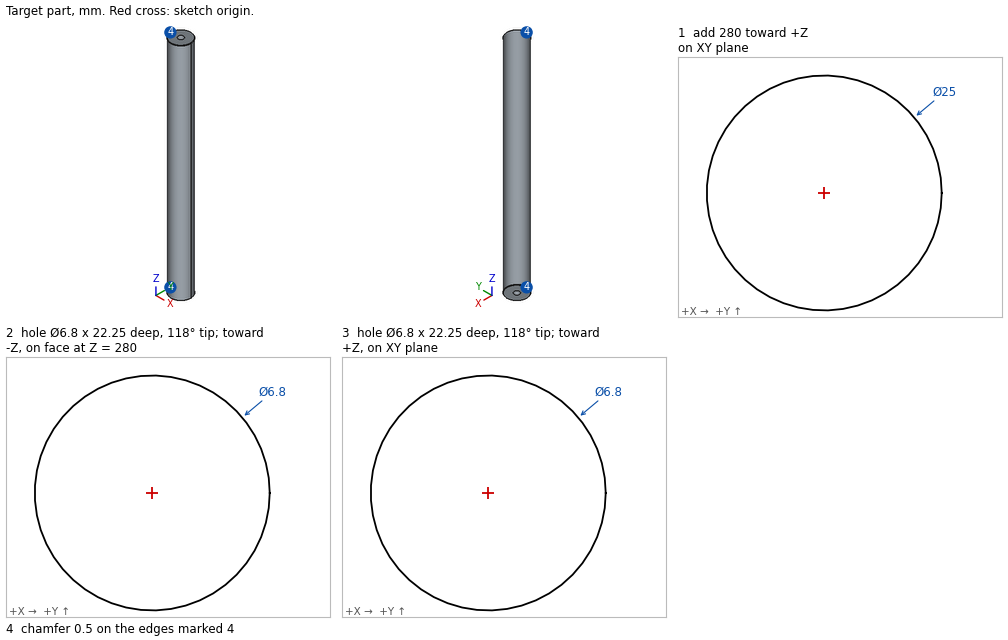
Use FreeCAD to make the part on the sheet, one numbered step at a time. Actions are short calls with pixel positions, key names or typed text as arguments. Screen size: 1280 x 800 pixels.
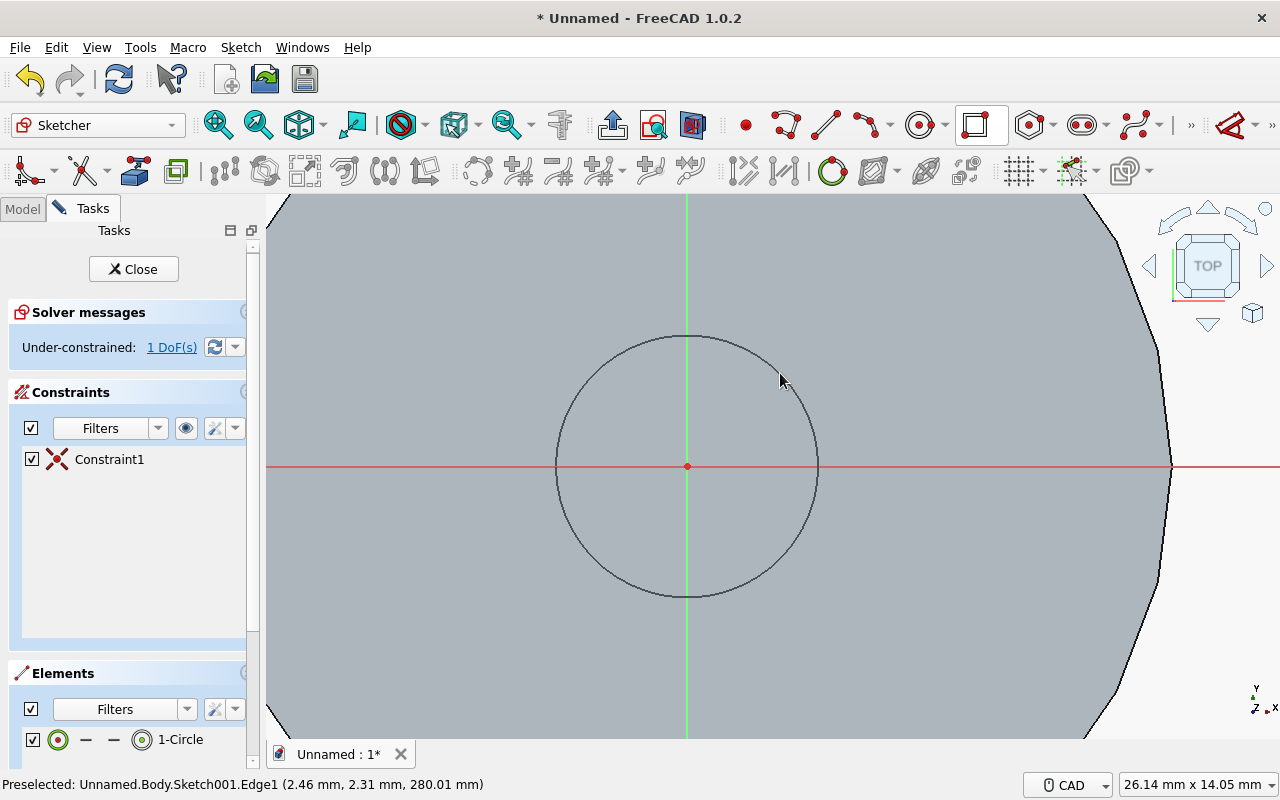
click(1230, 126)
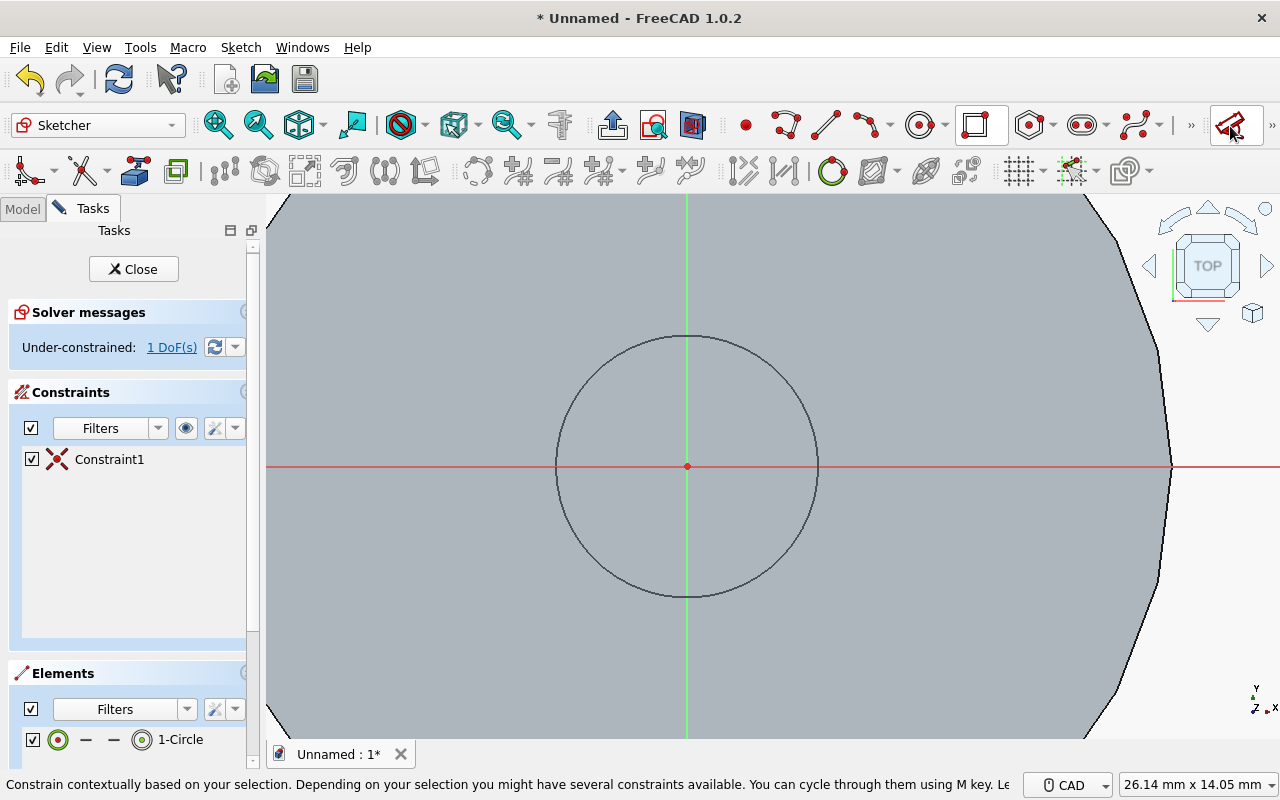
click(779, 373)
click(801, 350)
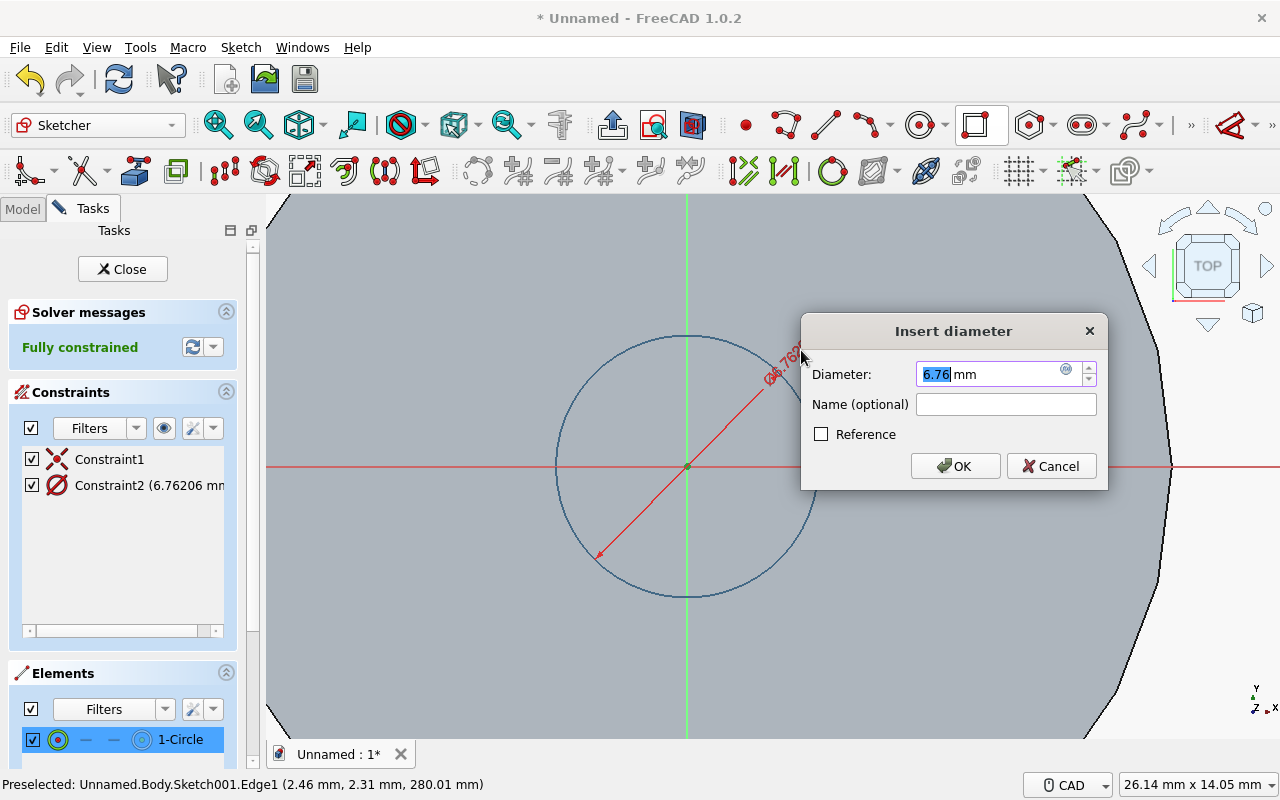
text(6.8)
key(Return)
key(Escape)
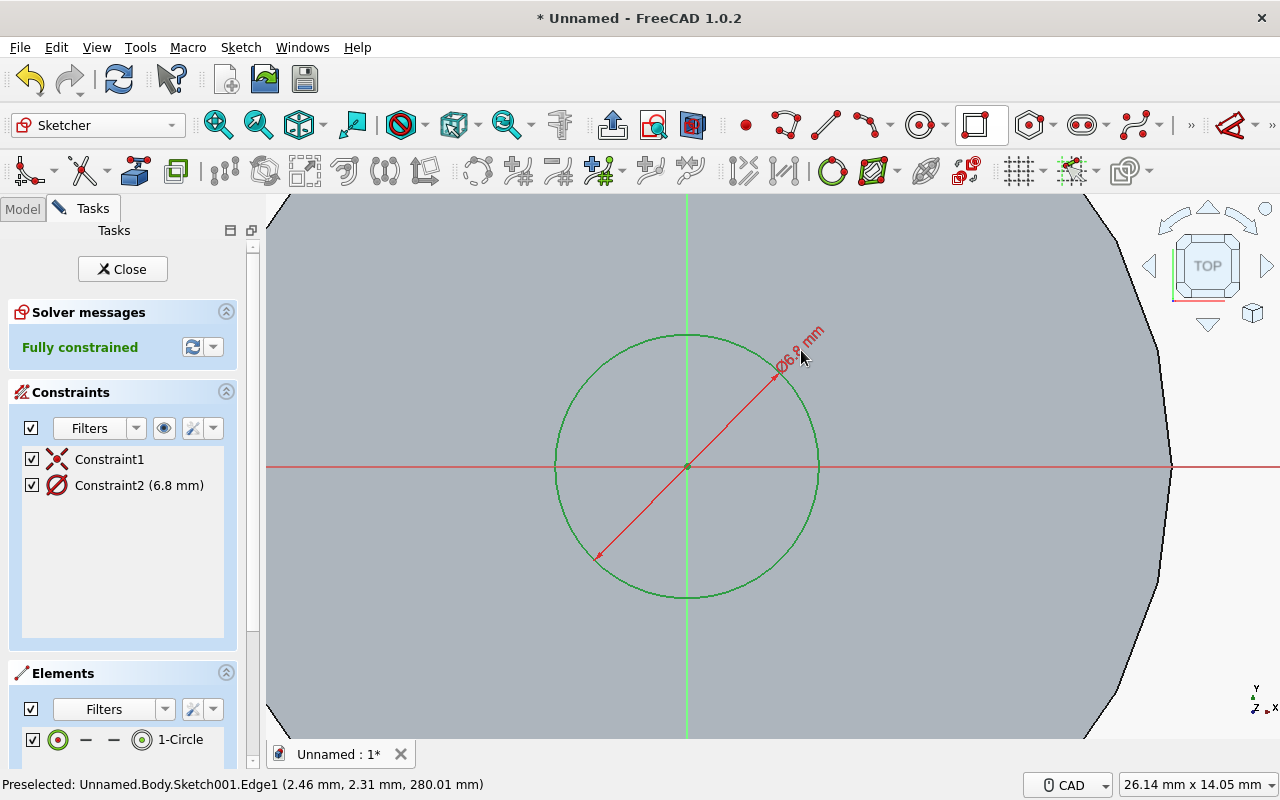
click(123, 269)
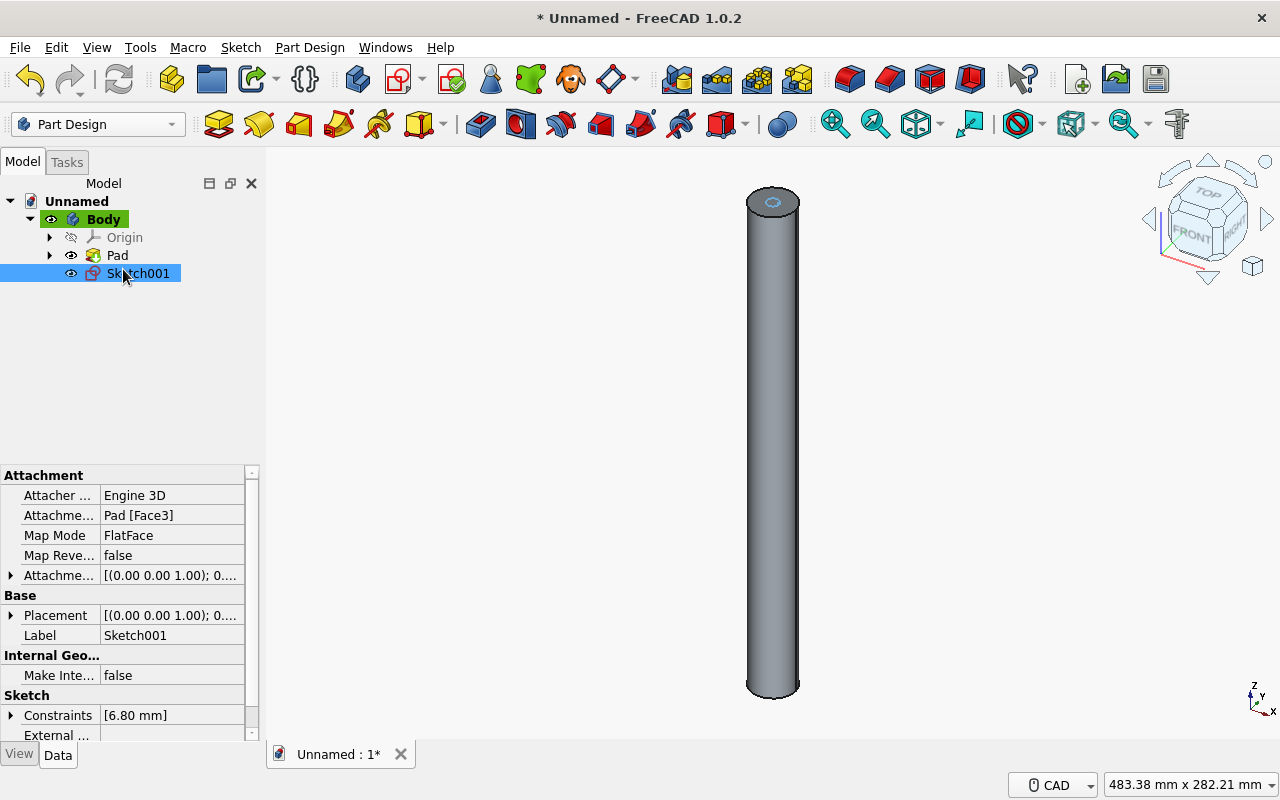
click(522, 124)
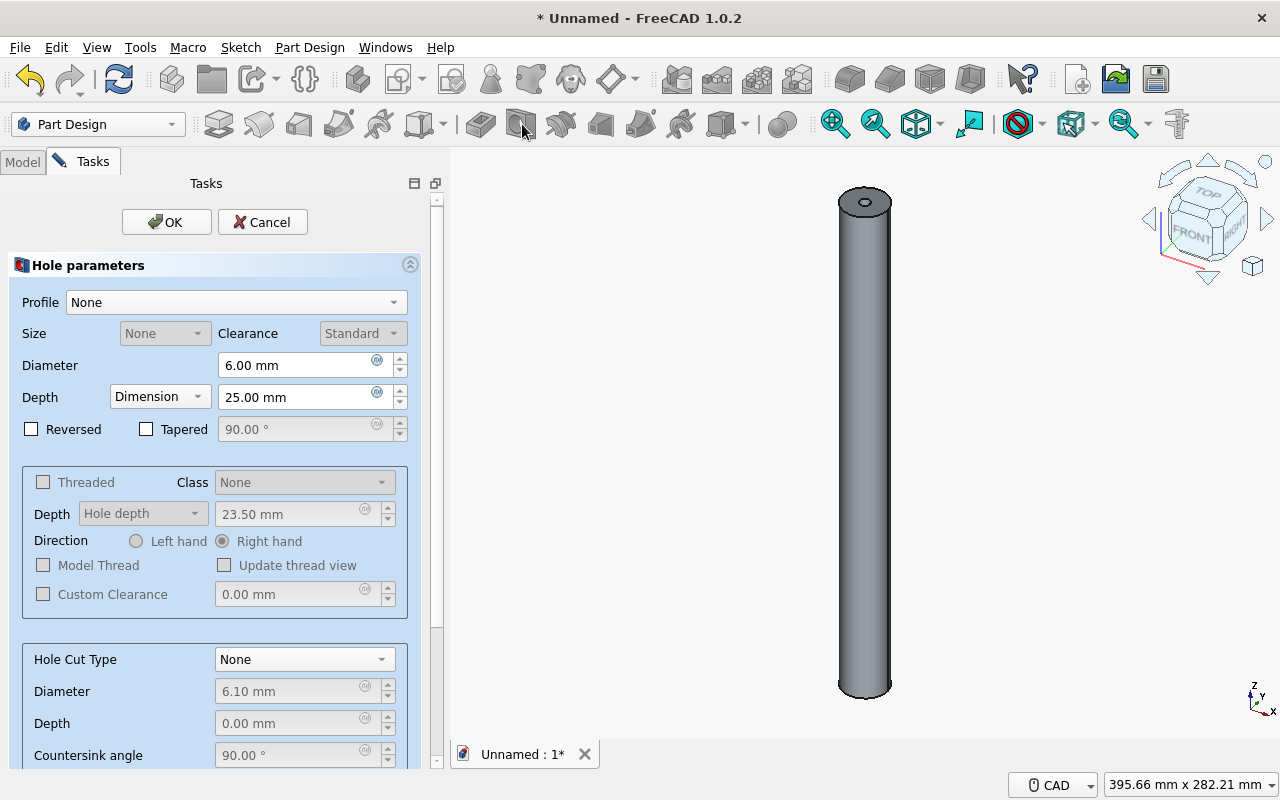
triple_click(305, 365)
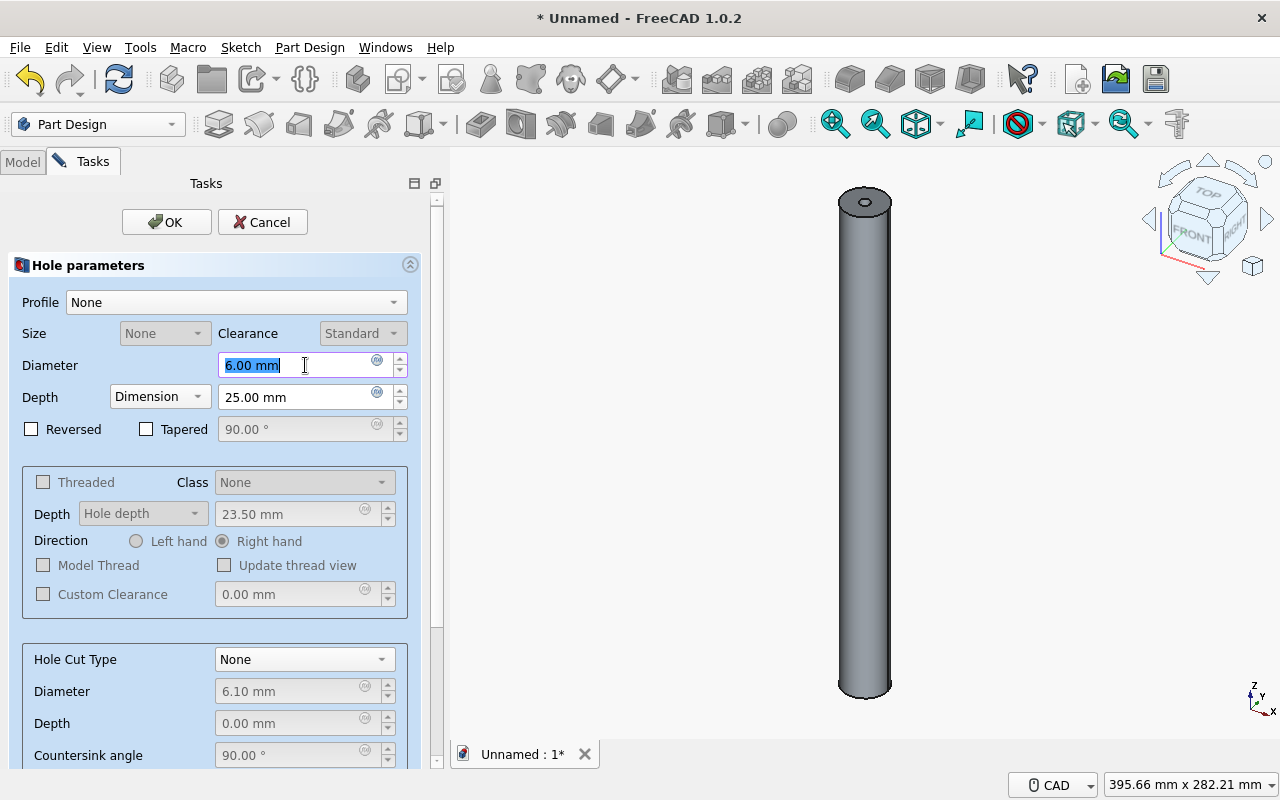
text(6.8)
key(Tab)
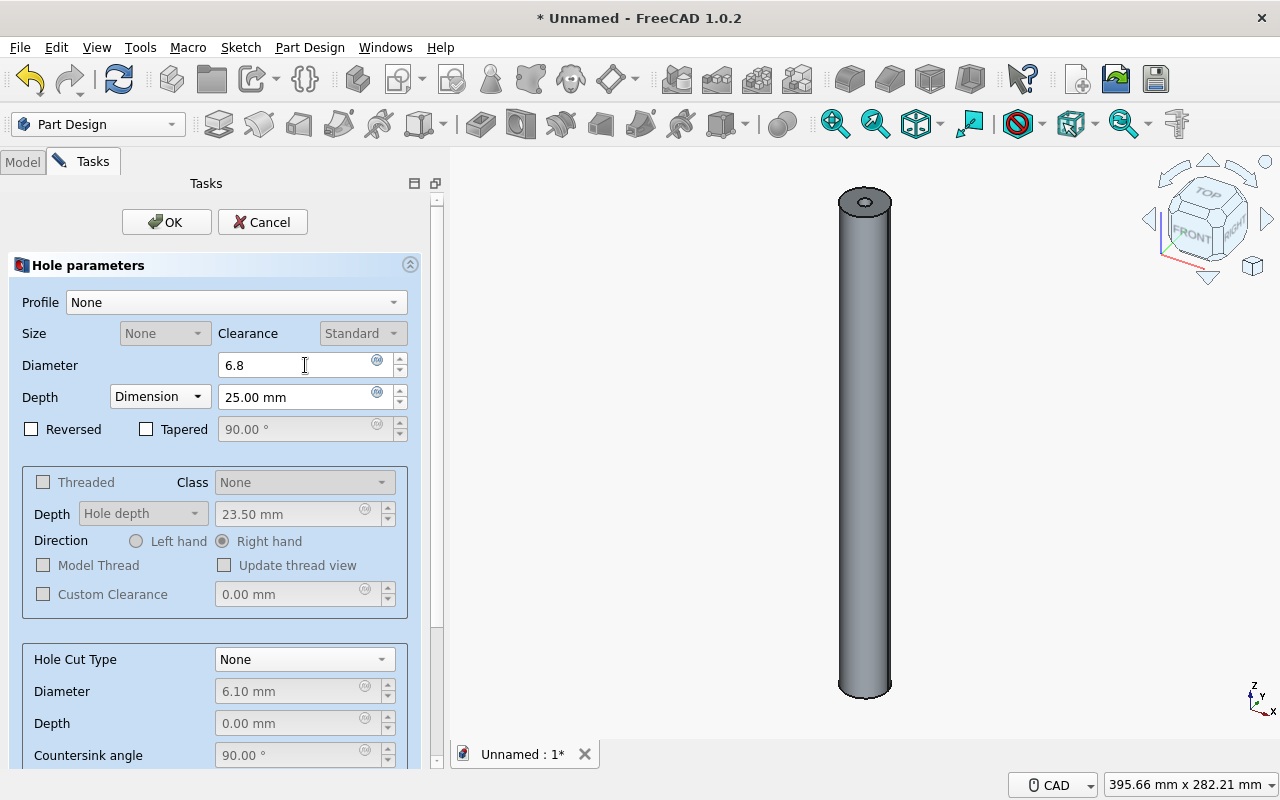
triple_click(305, 397)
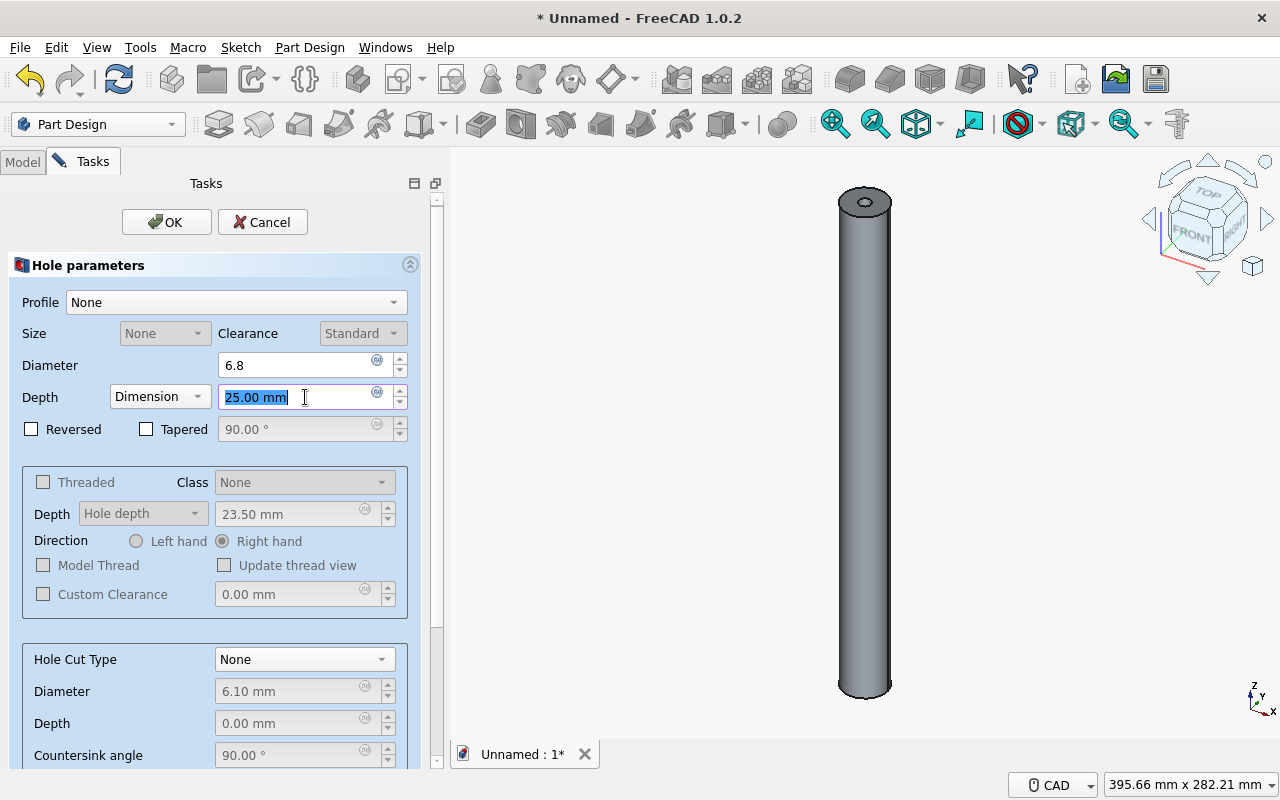
text(22.25)
key(Tab)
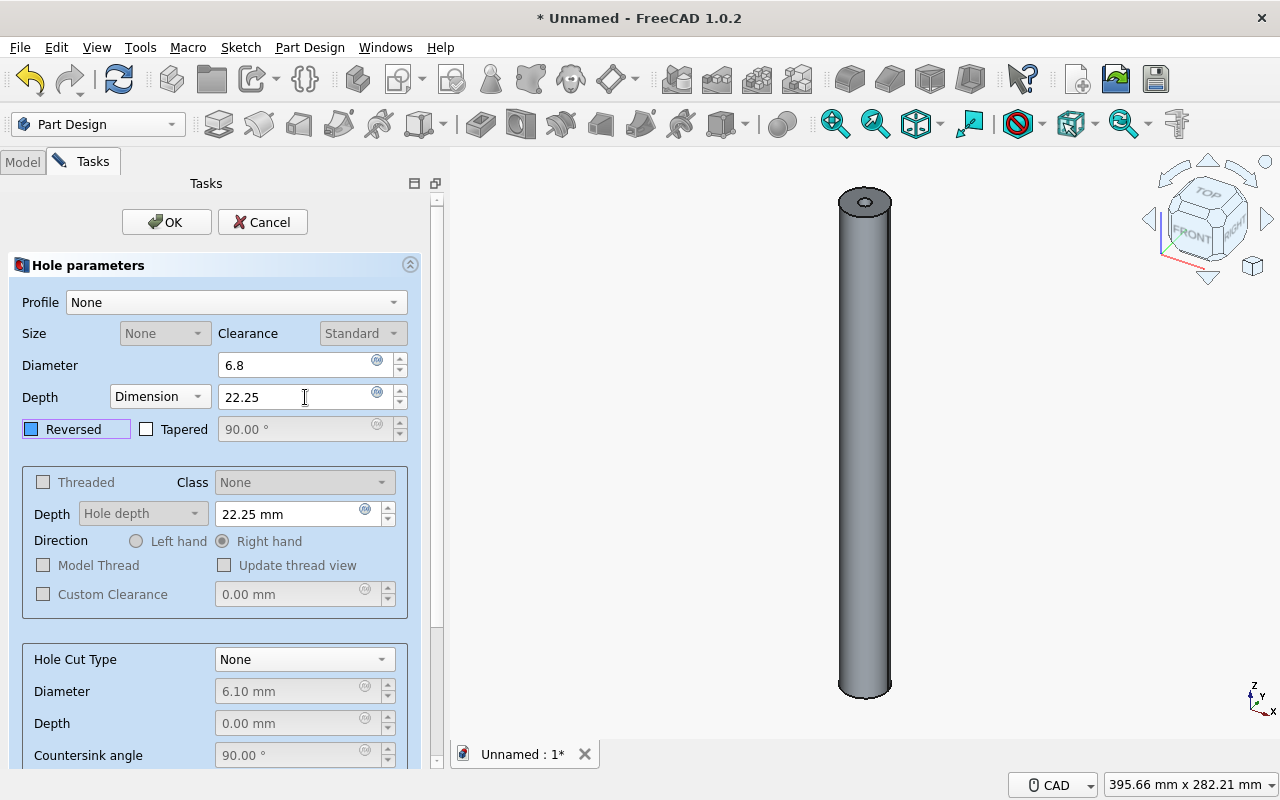
click(167, 222)